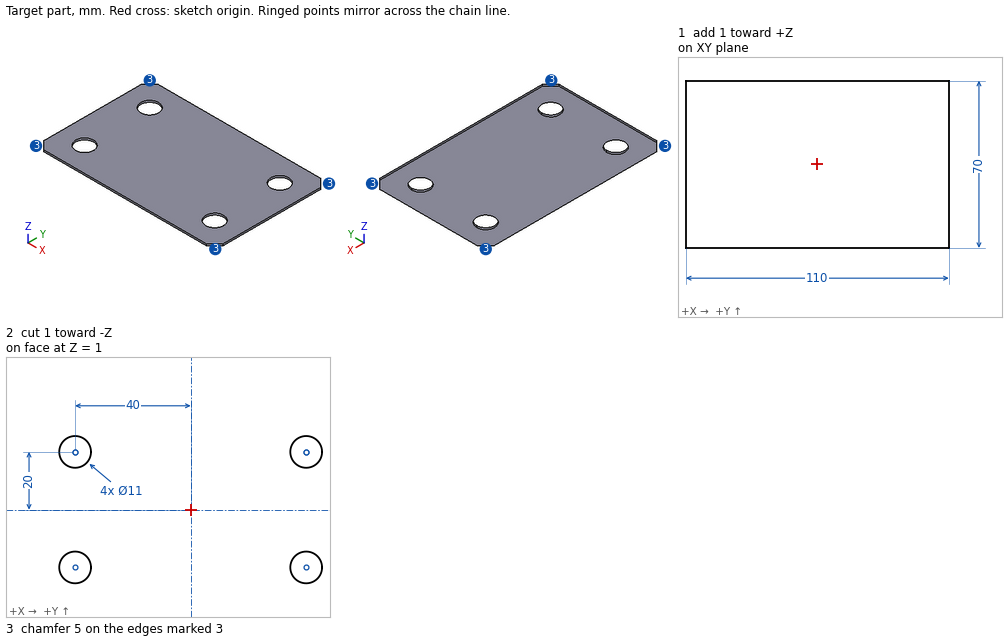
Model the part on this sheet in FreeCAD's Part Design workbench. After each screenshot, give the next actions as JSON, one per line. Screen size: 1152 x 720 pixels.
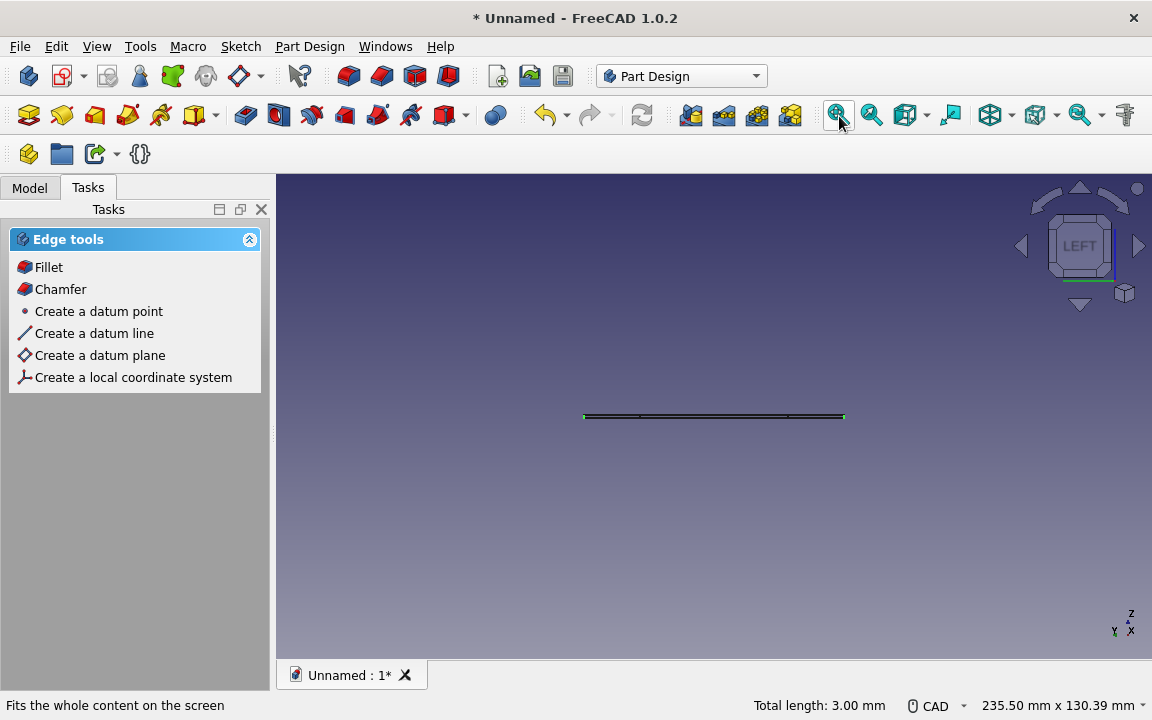
{"action": "key", "text": "0"}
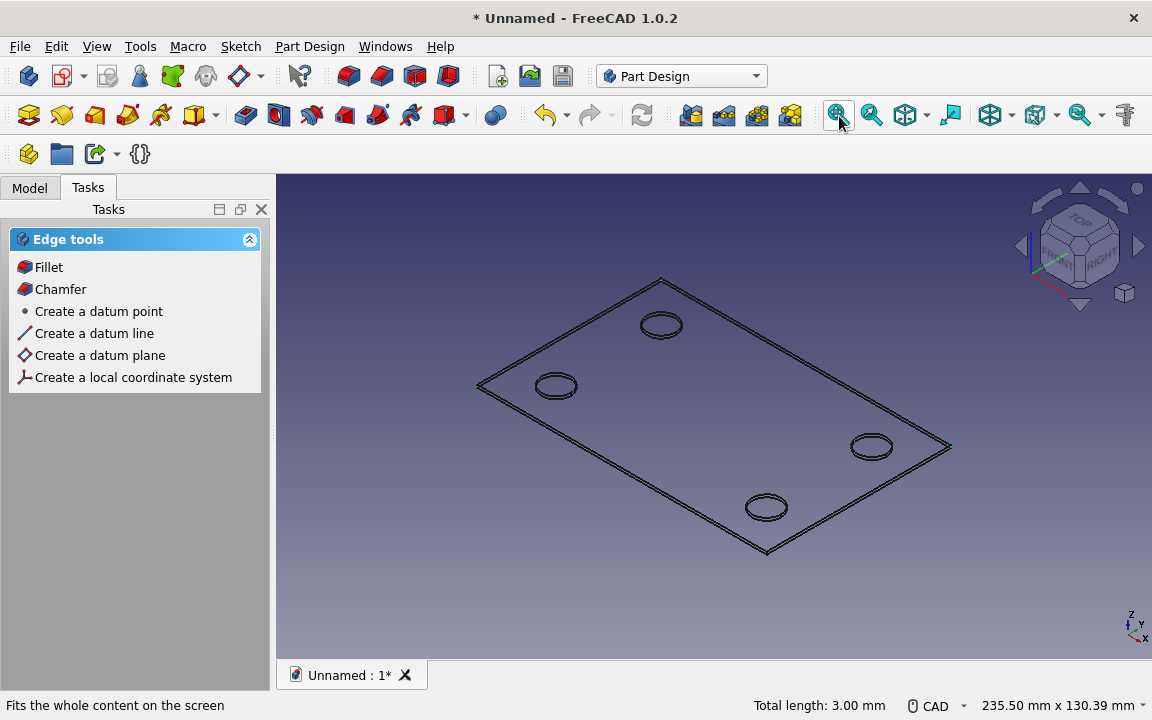
{"action": "scroll", "coordinate": [767, 552], "scroll_direction": "up", "scroll_amount": 12}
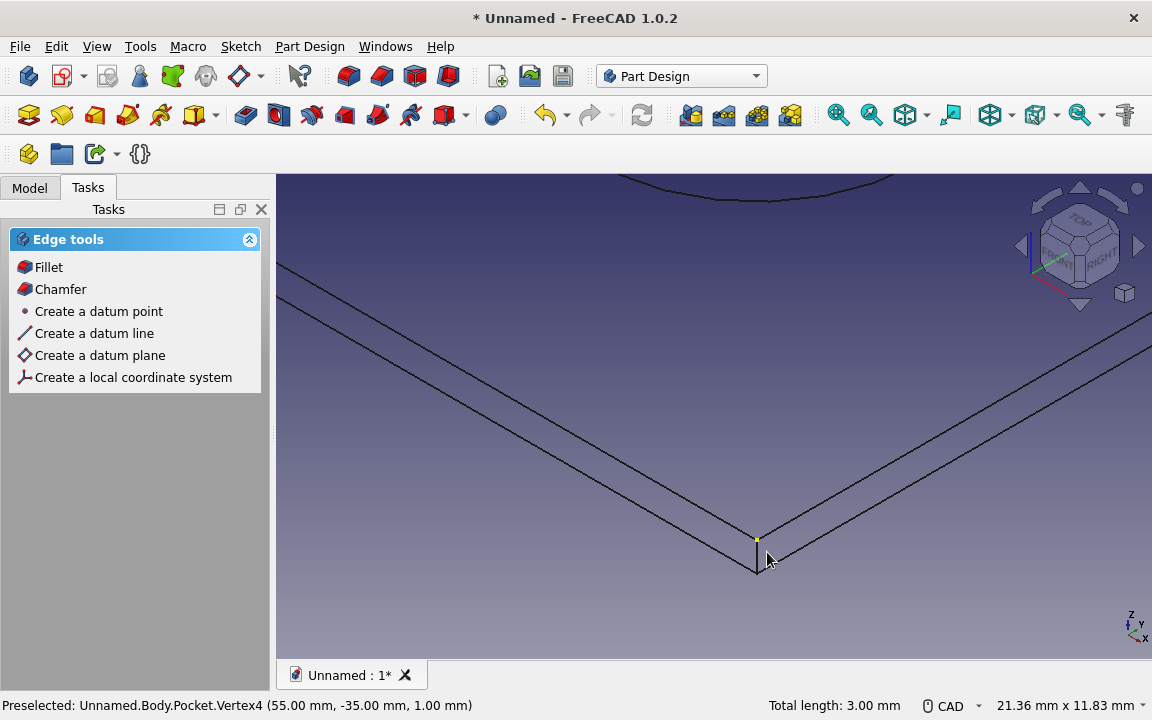
{"action": "left_click", "coordinate": [757, 556], "text": "ctrl"}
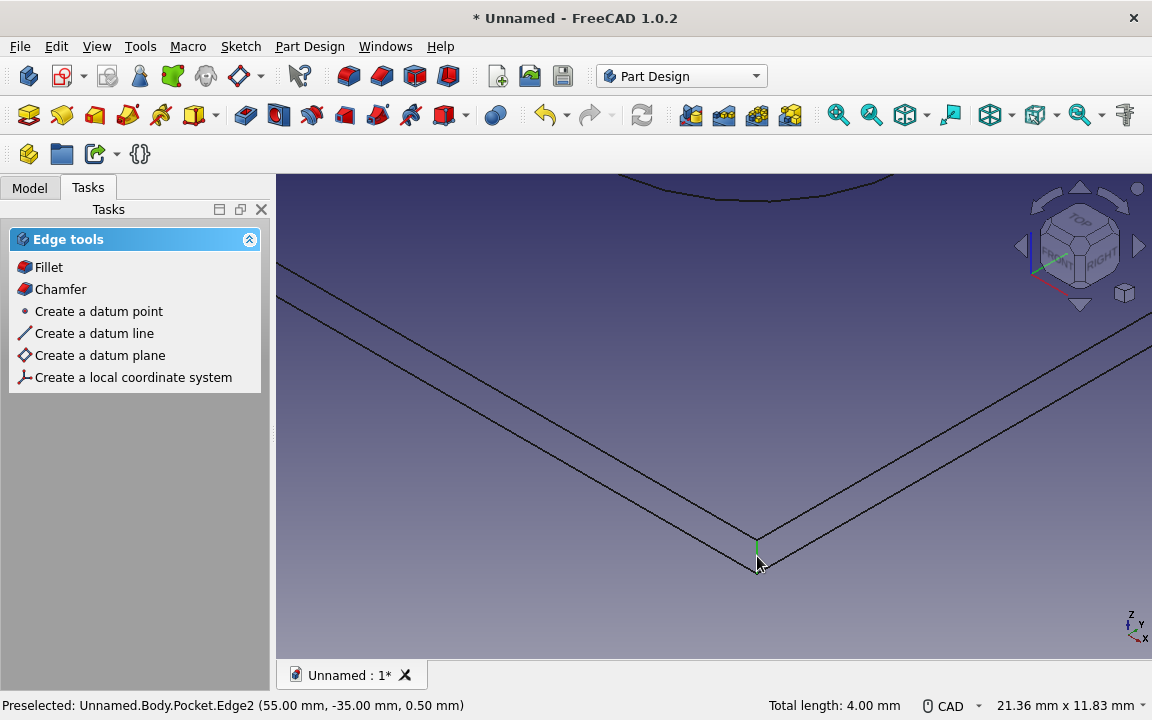
{"action": "key", "text": "v 1"}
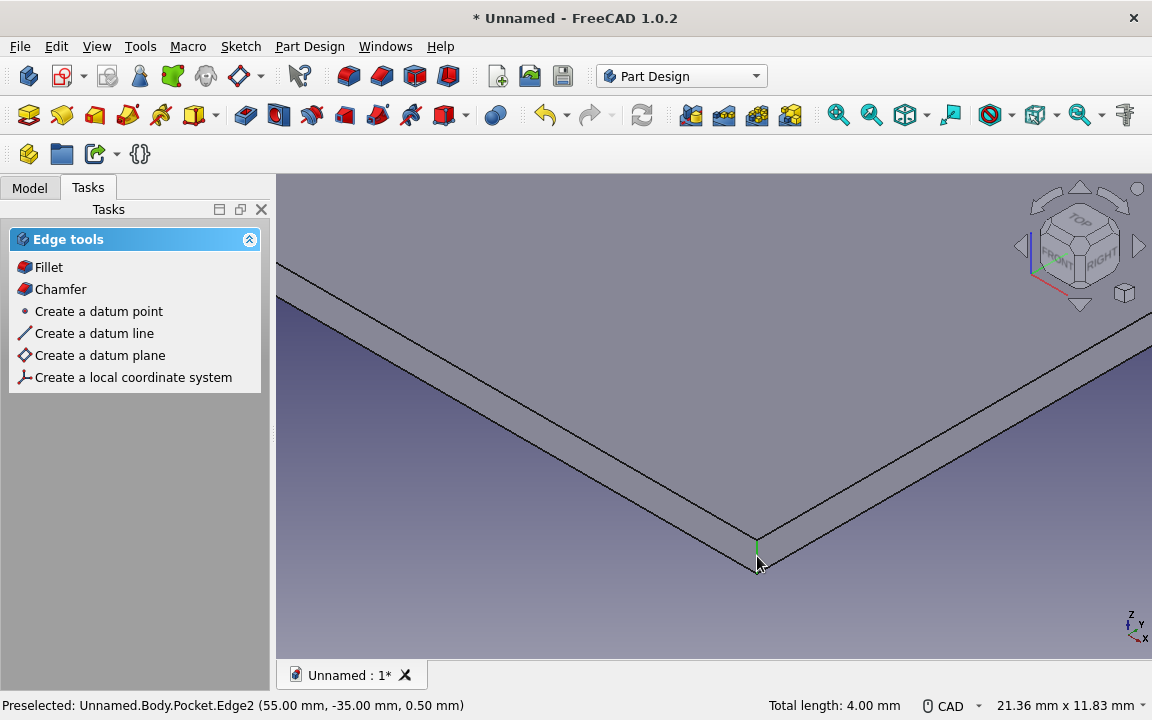
{"action": "left_click", "coordinate": [382, 76]}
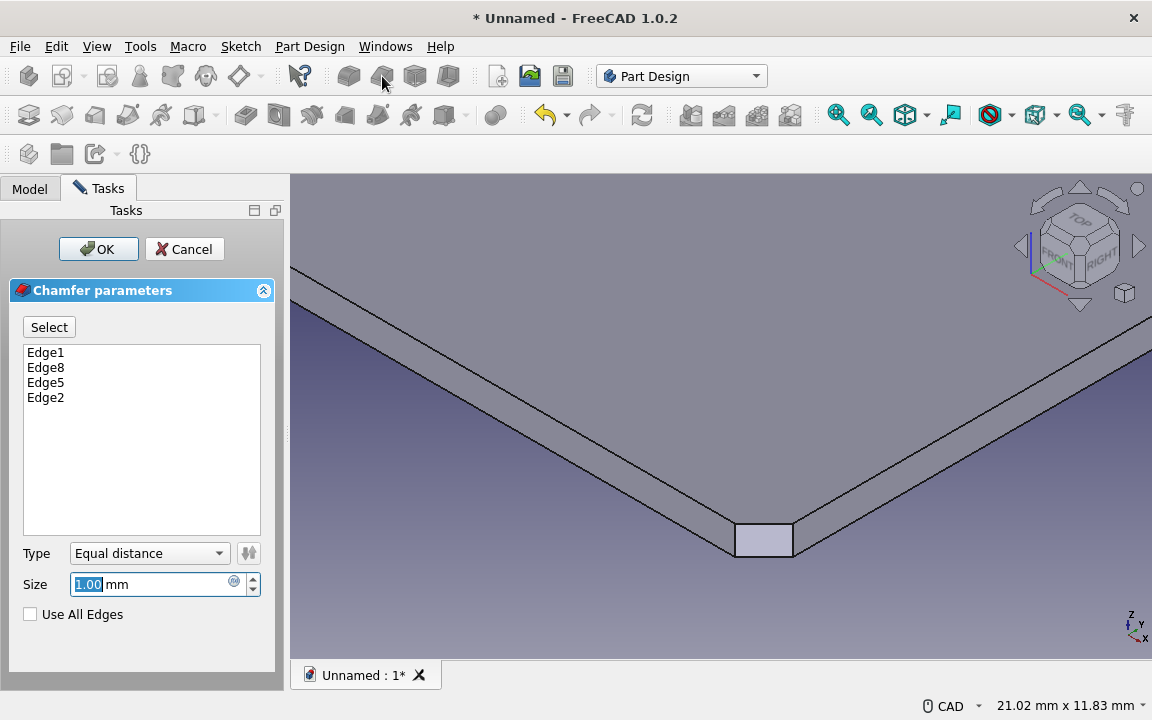
{"action": "type", "text": "5"}
{"action": "key", "text": "Tab"}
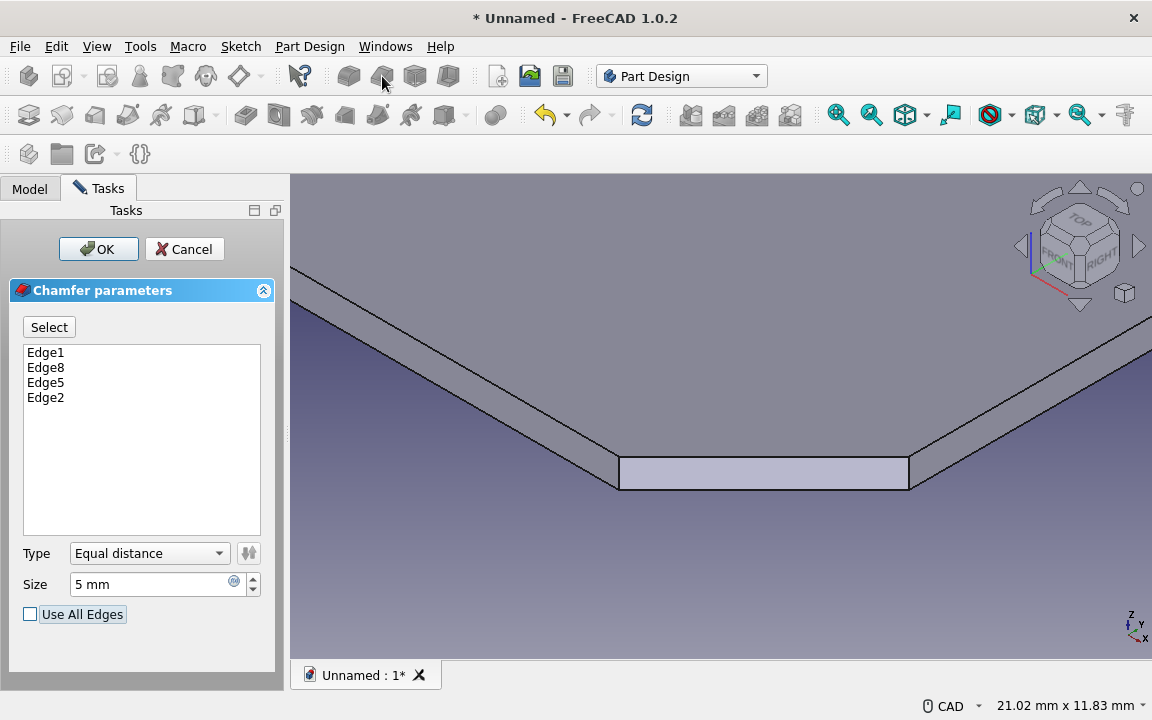
{"action": "left_click", "coordinate": [99, 249]}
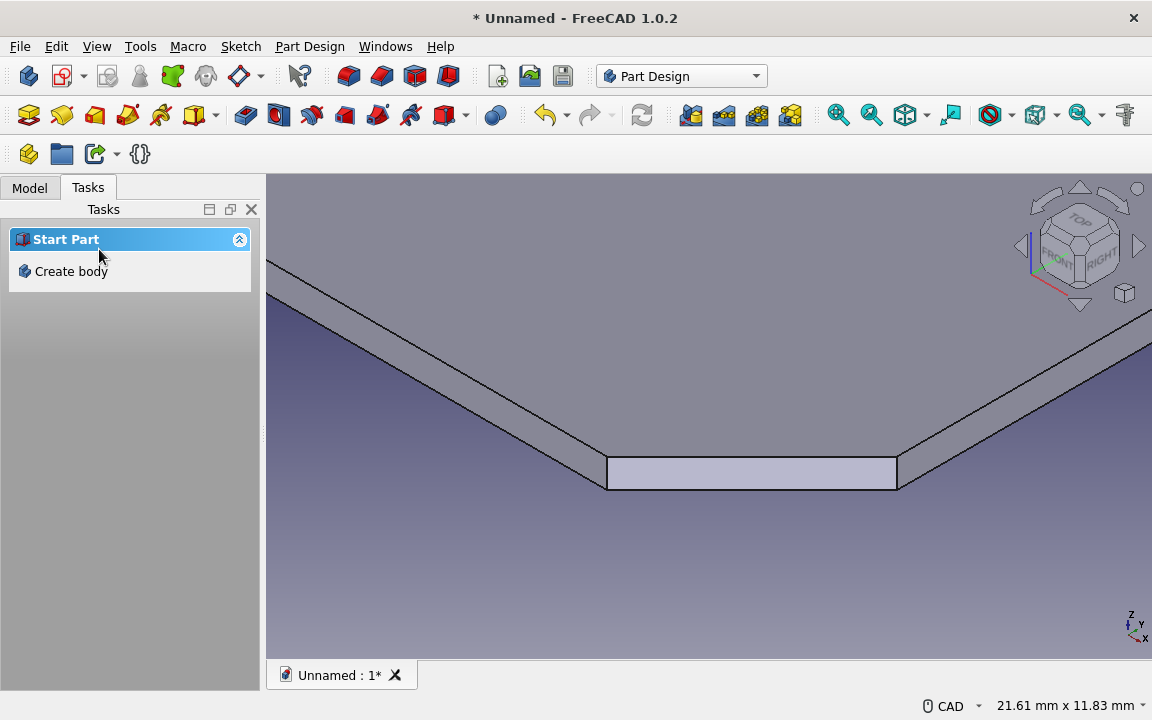
{"action": "left_click", "coordinate": [839, 116]}